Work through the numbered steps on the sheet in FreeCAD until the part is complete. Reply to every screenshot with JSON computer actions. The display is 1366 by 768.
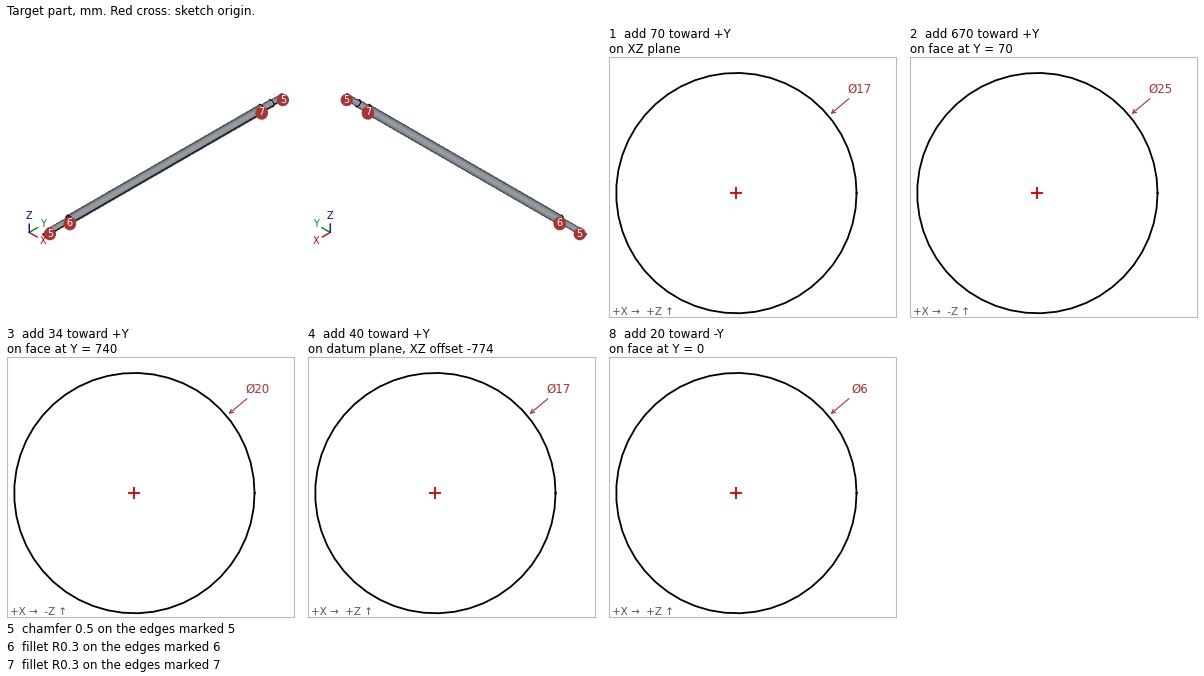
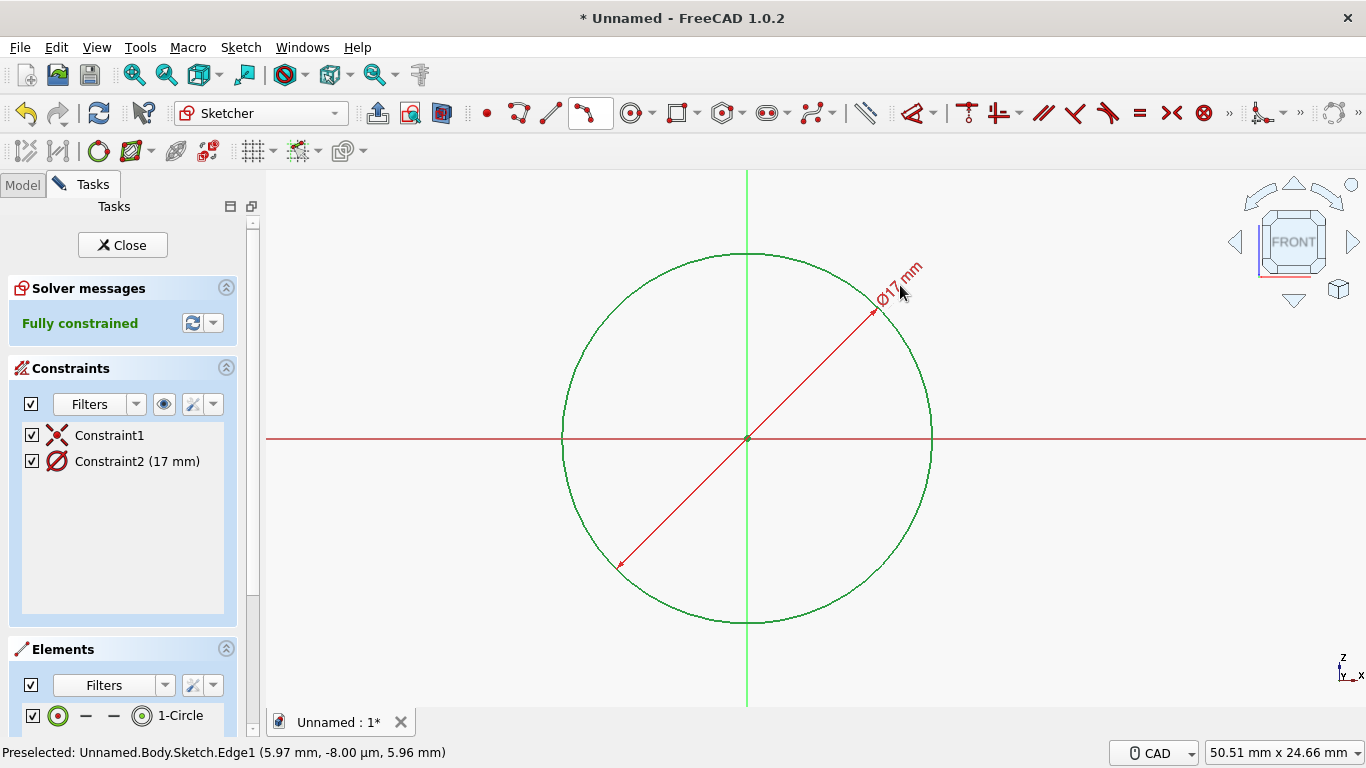
{"action": "left_click", "coordinate": [123, 245]}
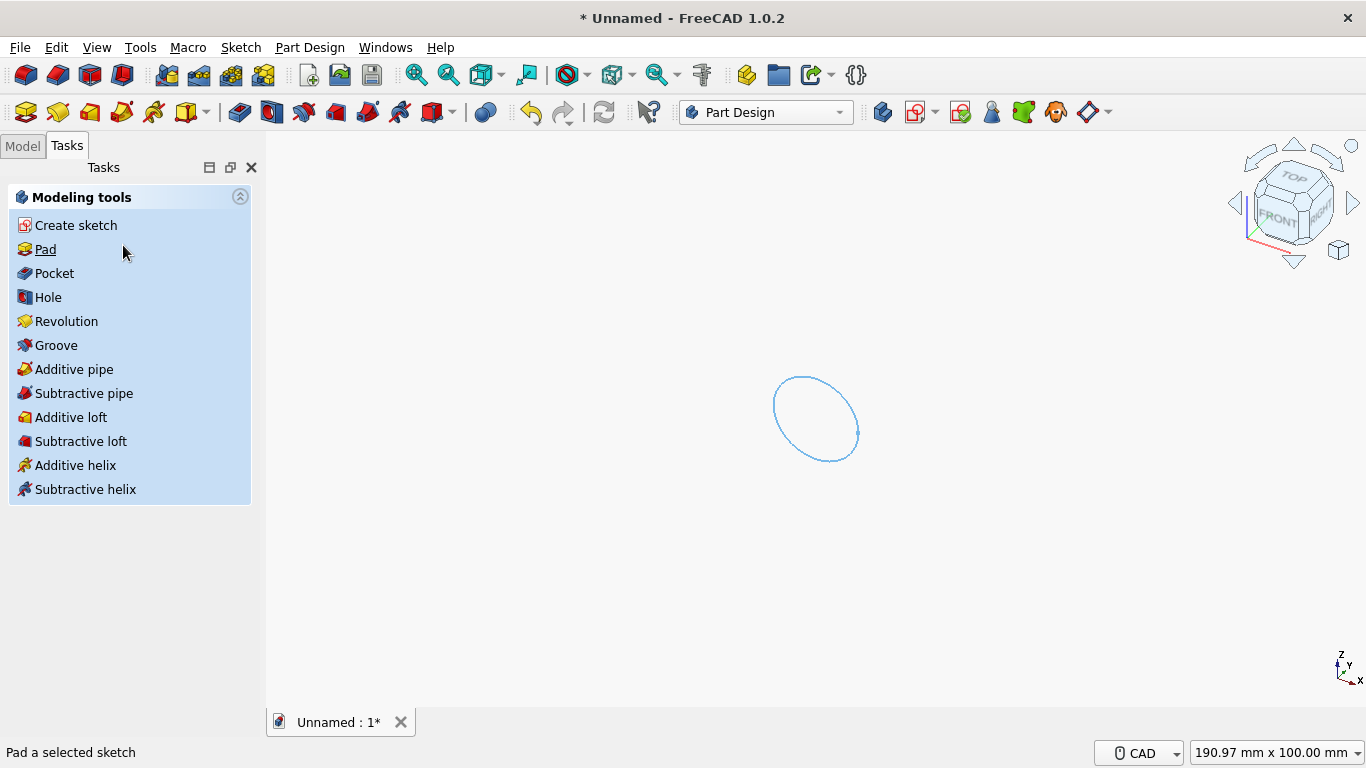
{"action": "left_click", "coordinate": [26, 112]}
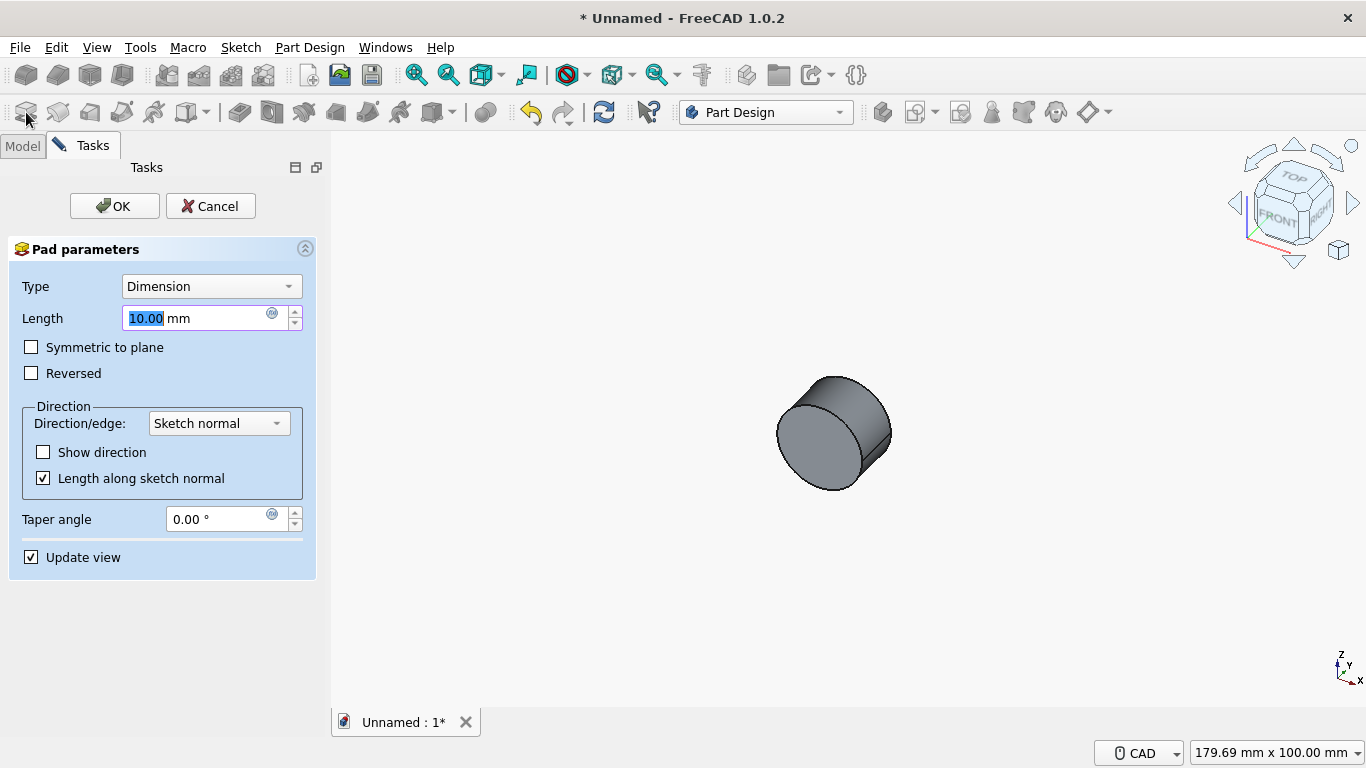
{"action": "type", "text": "70"}
{"action": "key", "text": "Tab"}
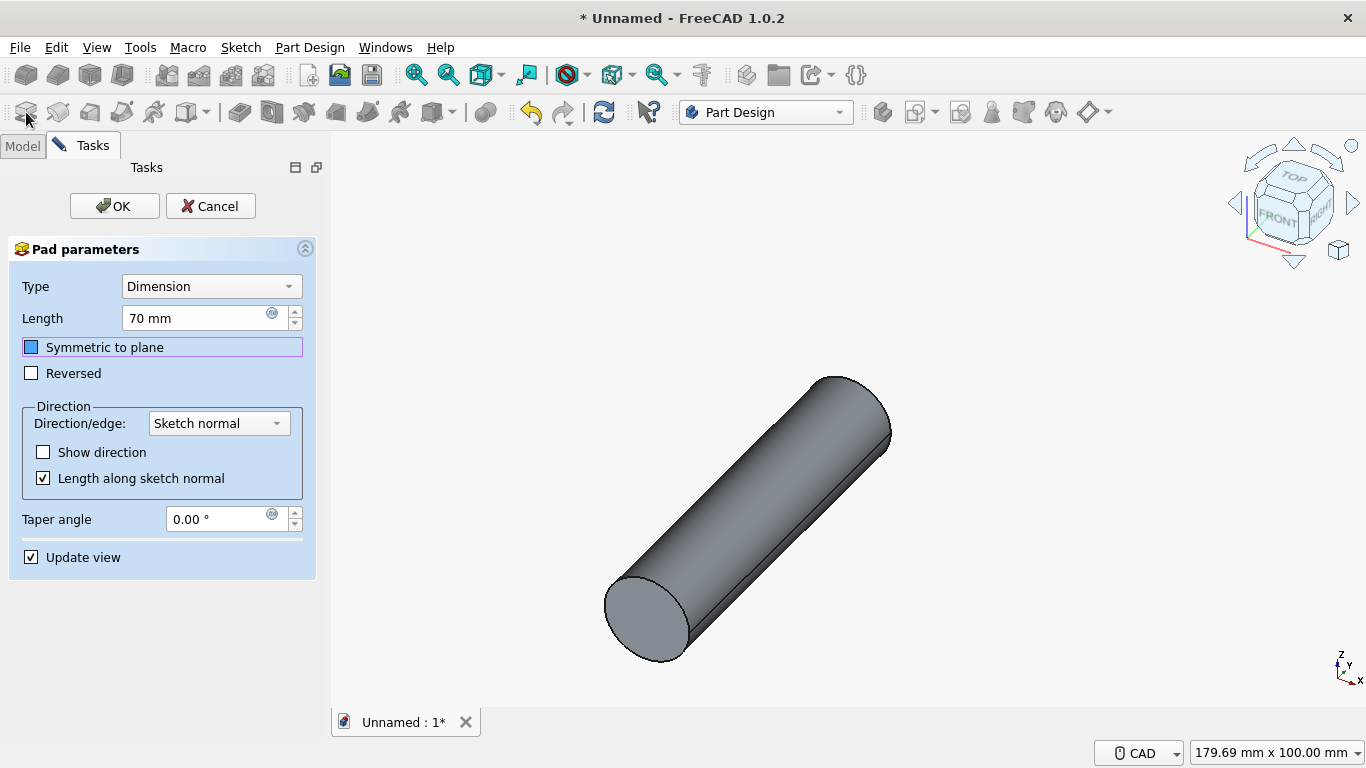
{"action": "left_click", "coordinate": [30, 373]}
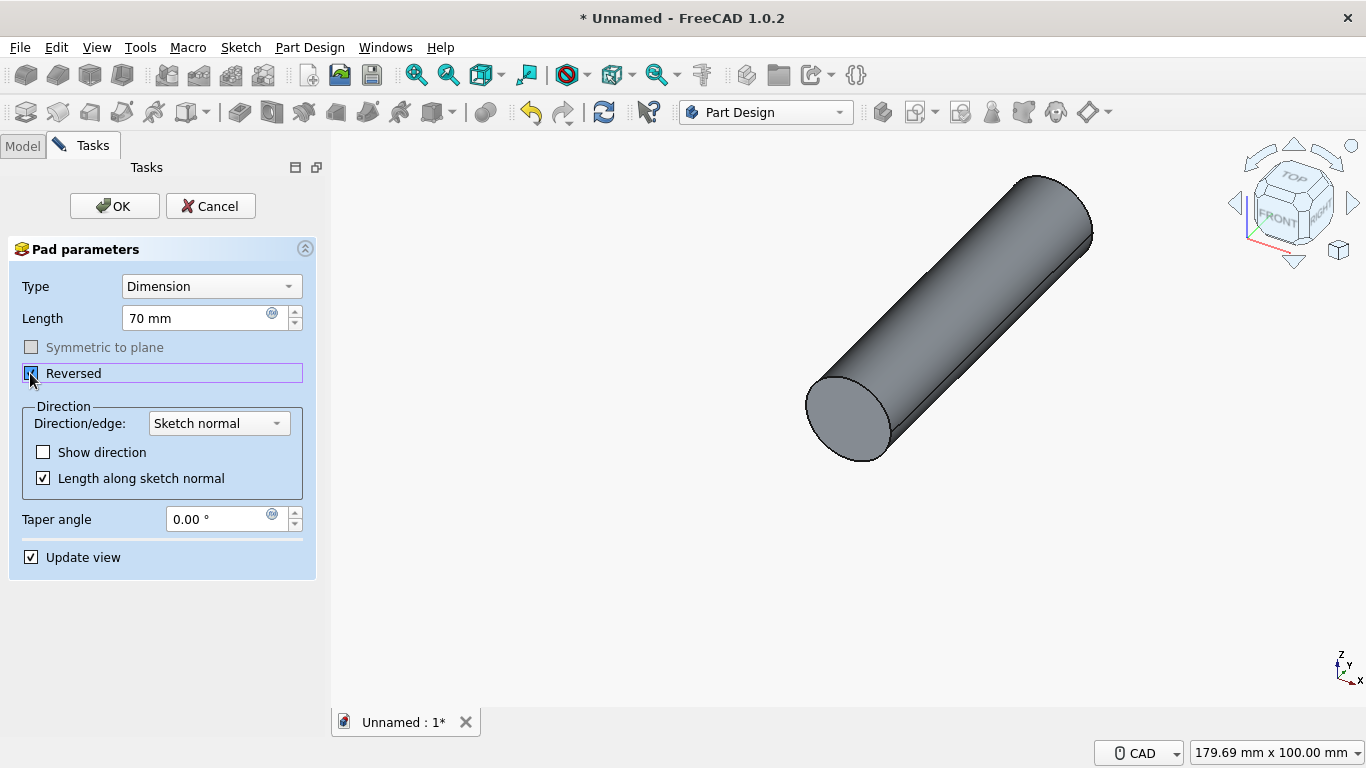
{"action": "left_click", "coordinate": [115, 206]}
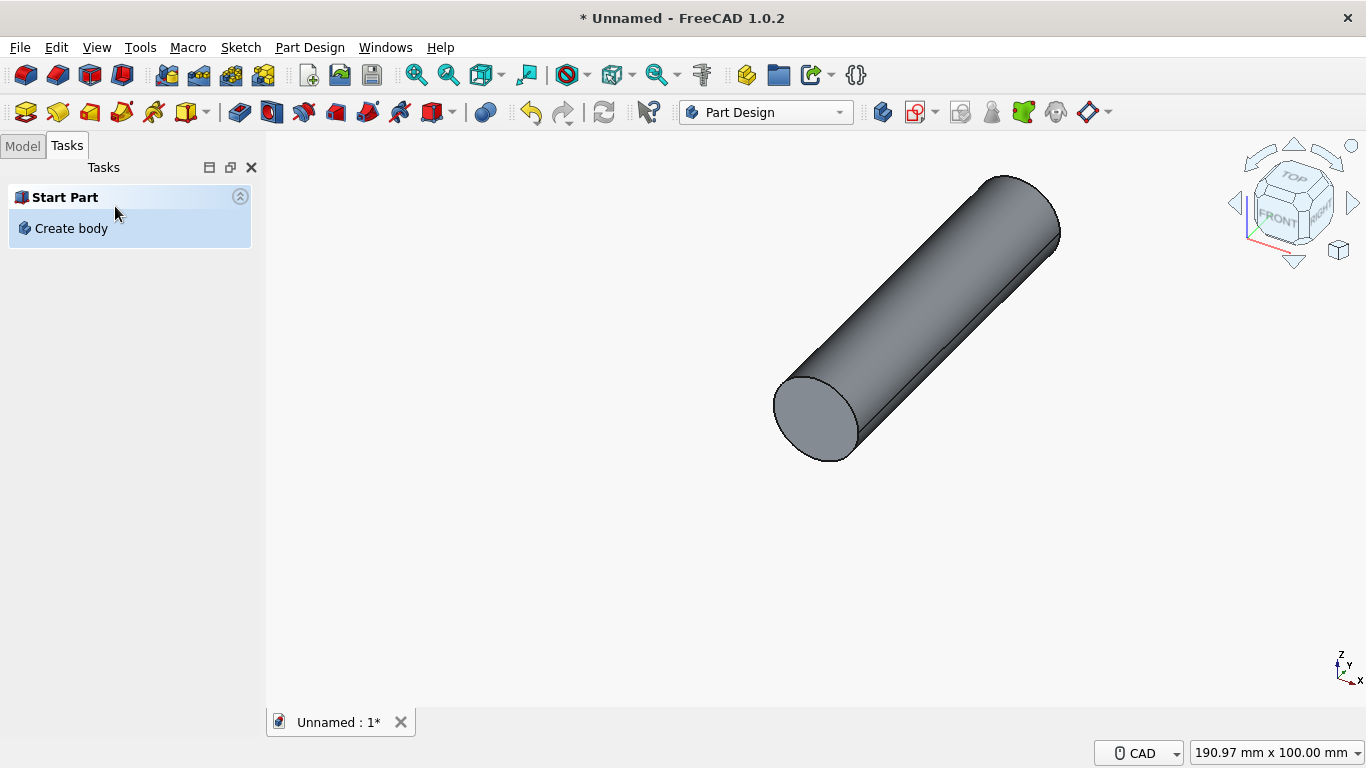
{"action": "key", "text": "4"}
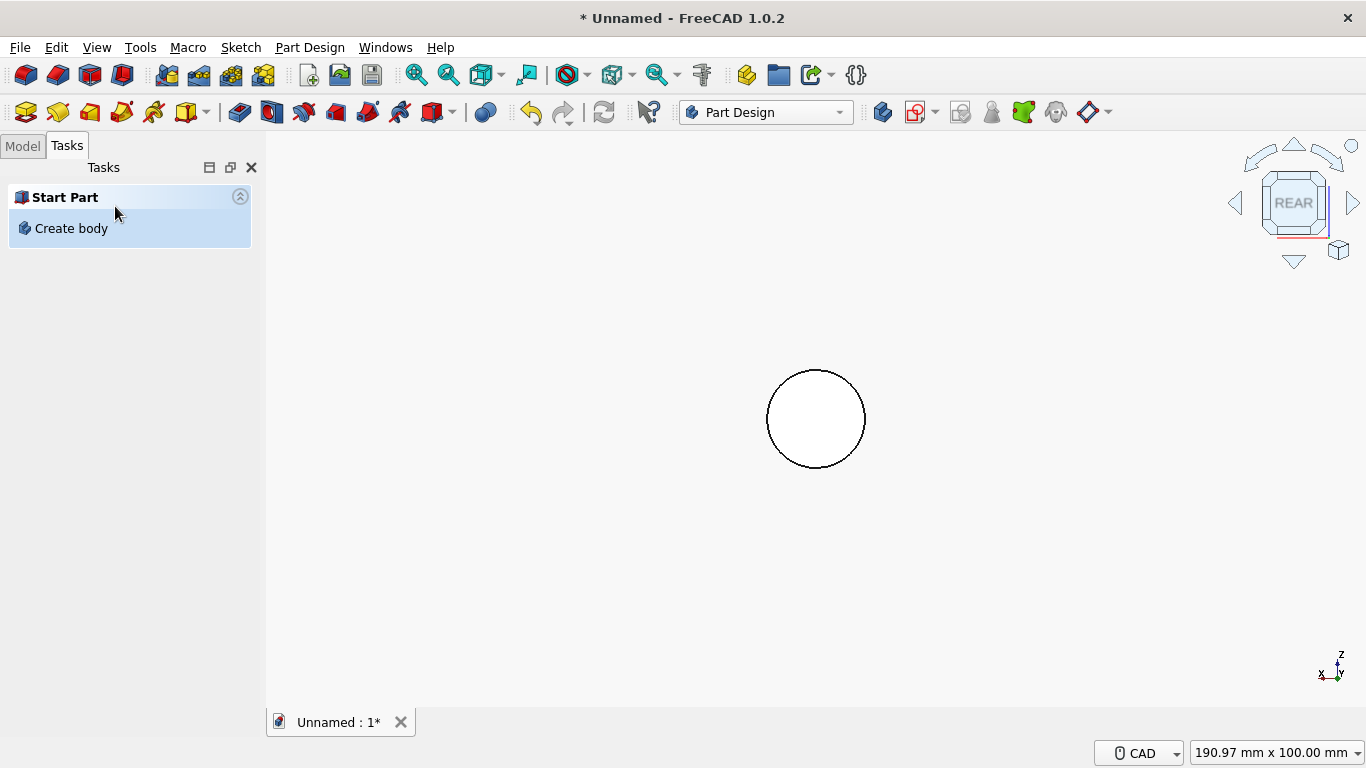
{"action": "key", "text": "v f"}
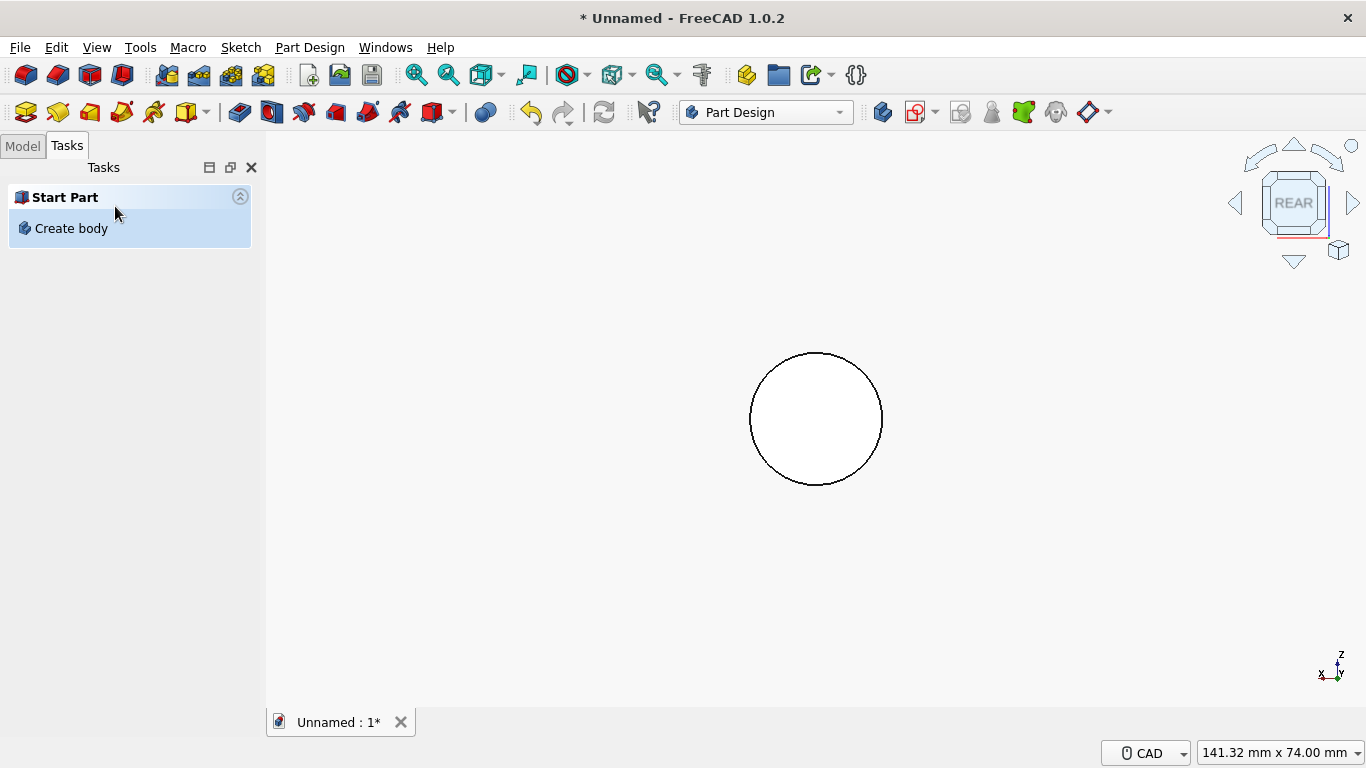
{"action": "left_click", "coordinate": [816, 418]}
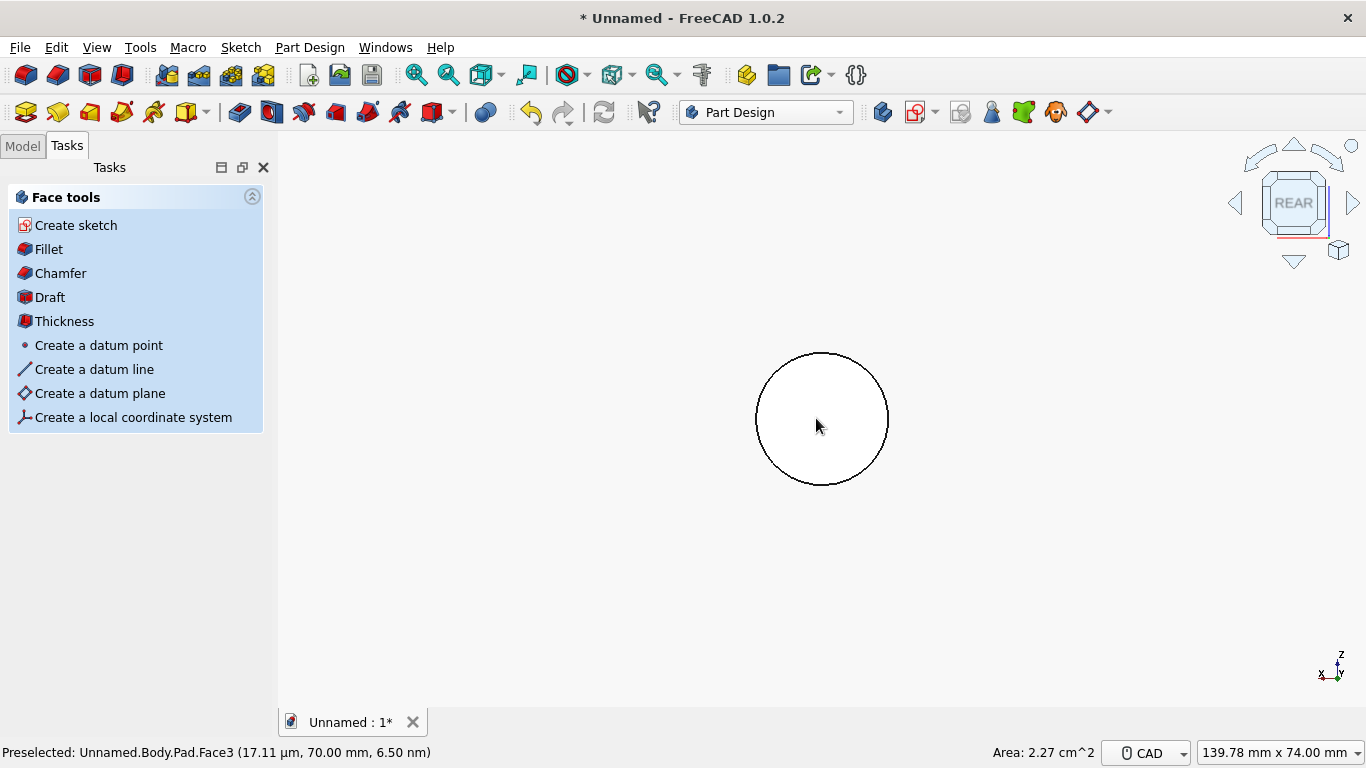
{"action": "left_click", "coordinate": [916, 112]}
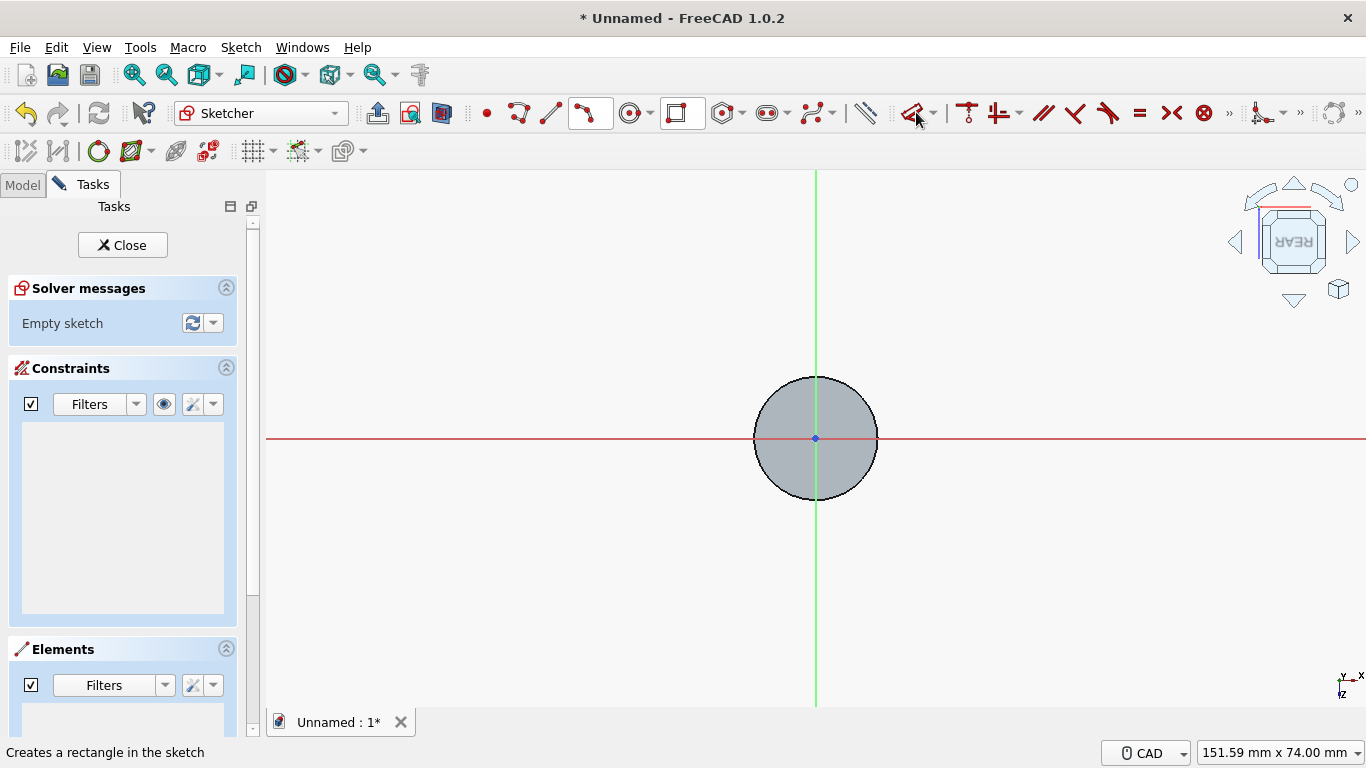
{"action": "scroll", "coordinate": [899, 438], "scroll_direction": "up", "scroll_amount": 3}